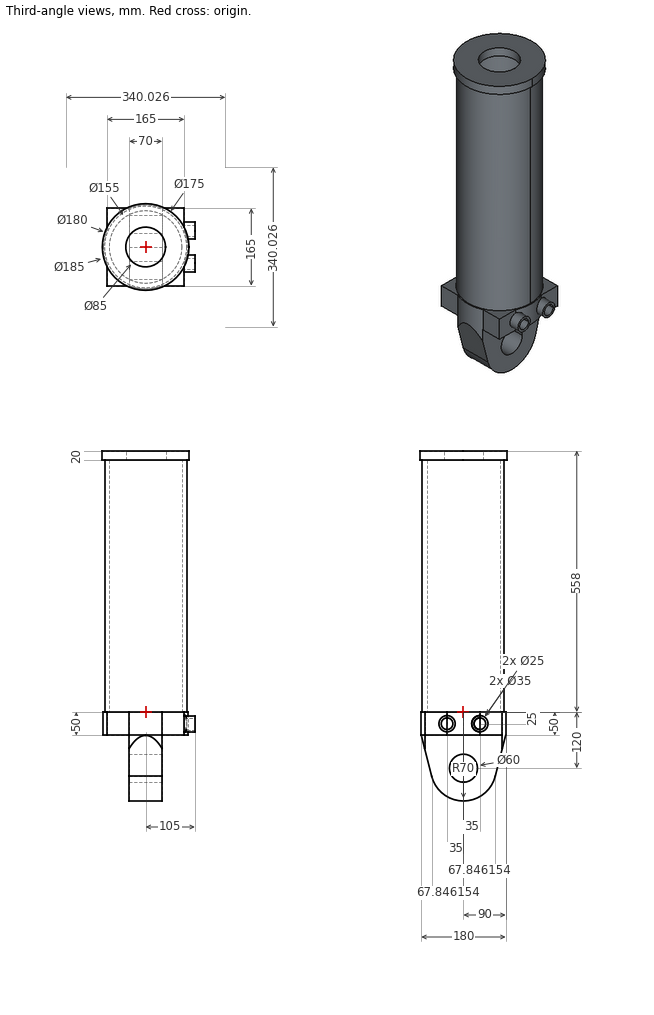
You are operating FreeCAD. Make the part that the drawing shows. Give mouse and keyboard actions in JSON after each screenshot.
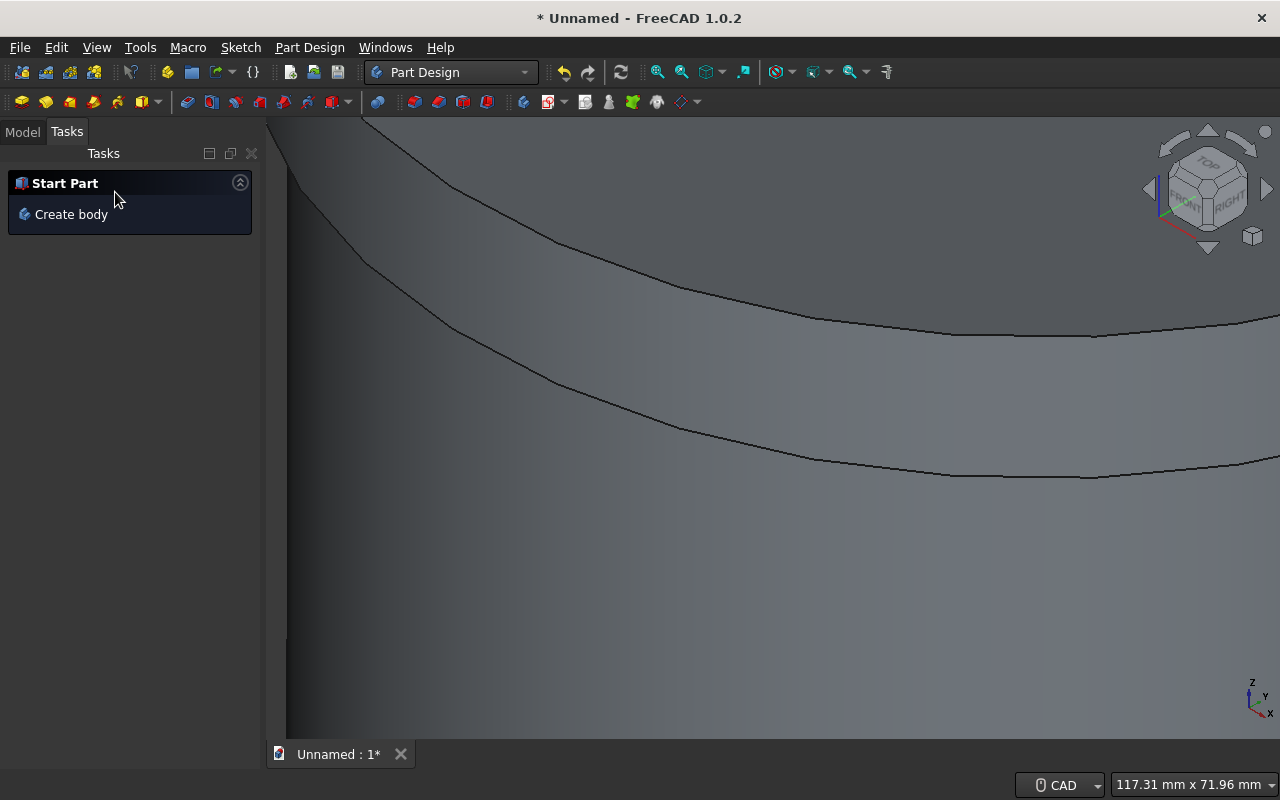
{"action": "left_click", "coordinate": [658, 72]}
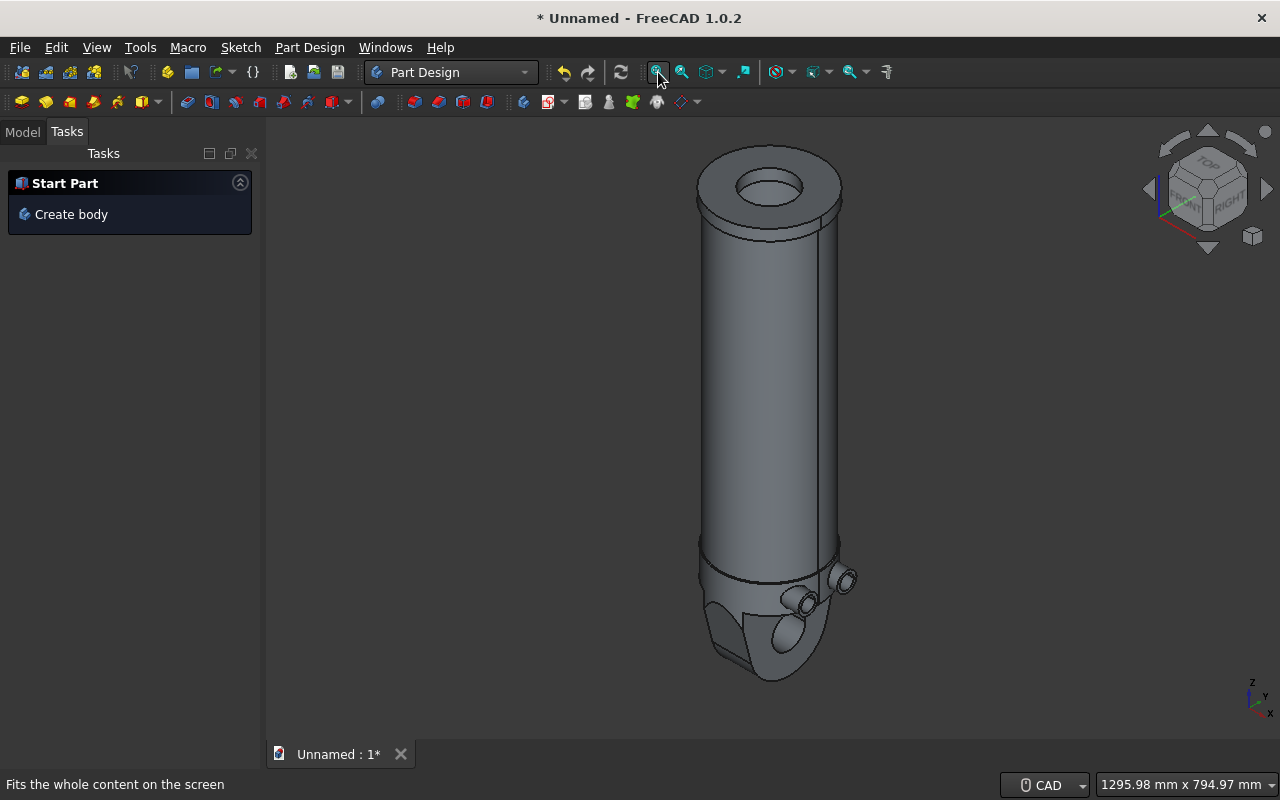
{"action": "key", "text": "5"}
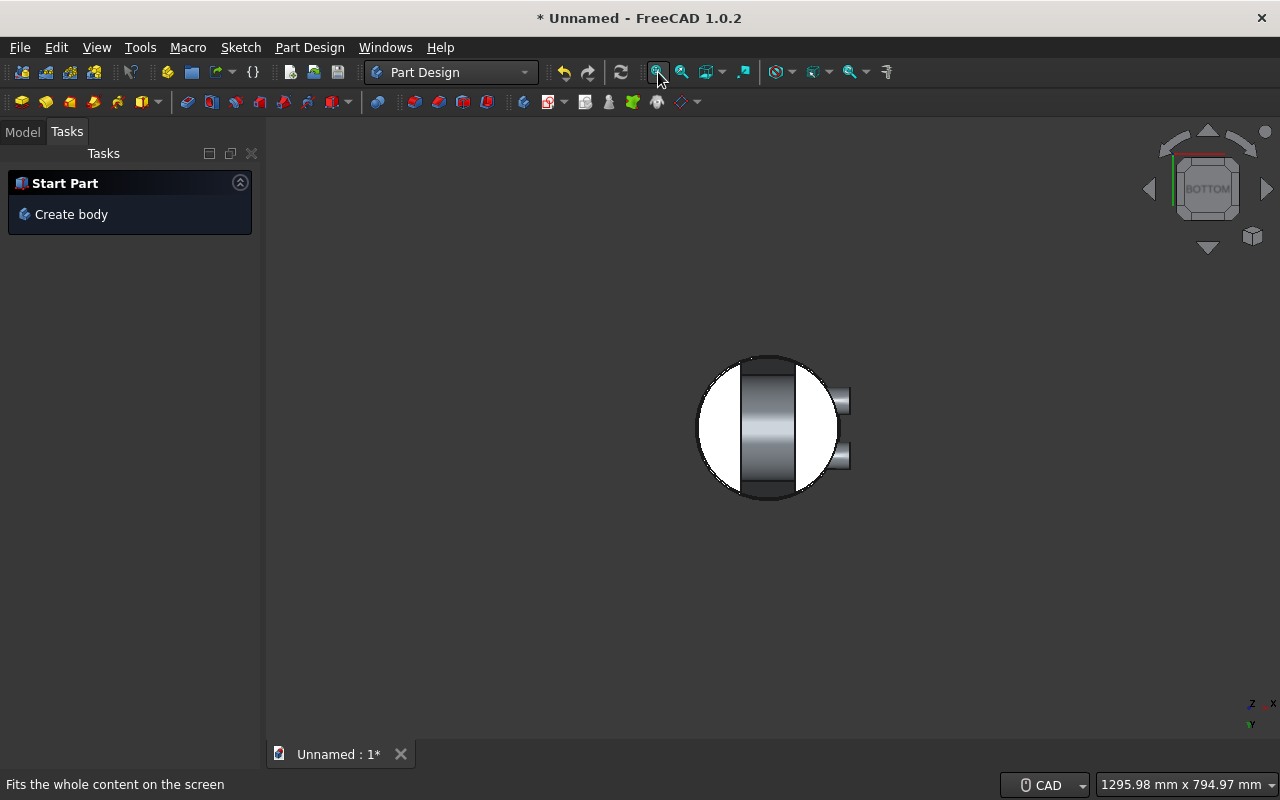
{"action": "left_click", "coordinate": [658, 72]}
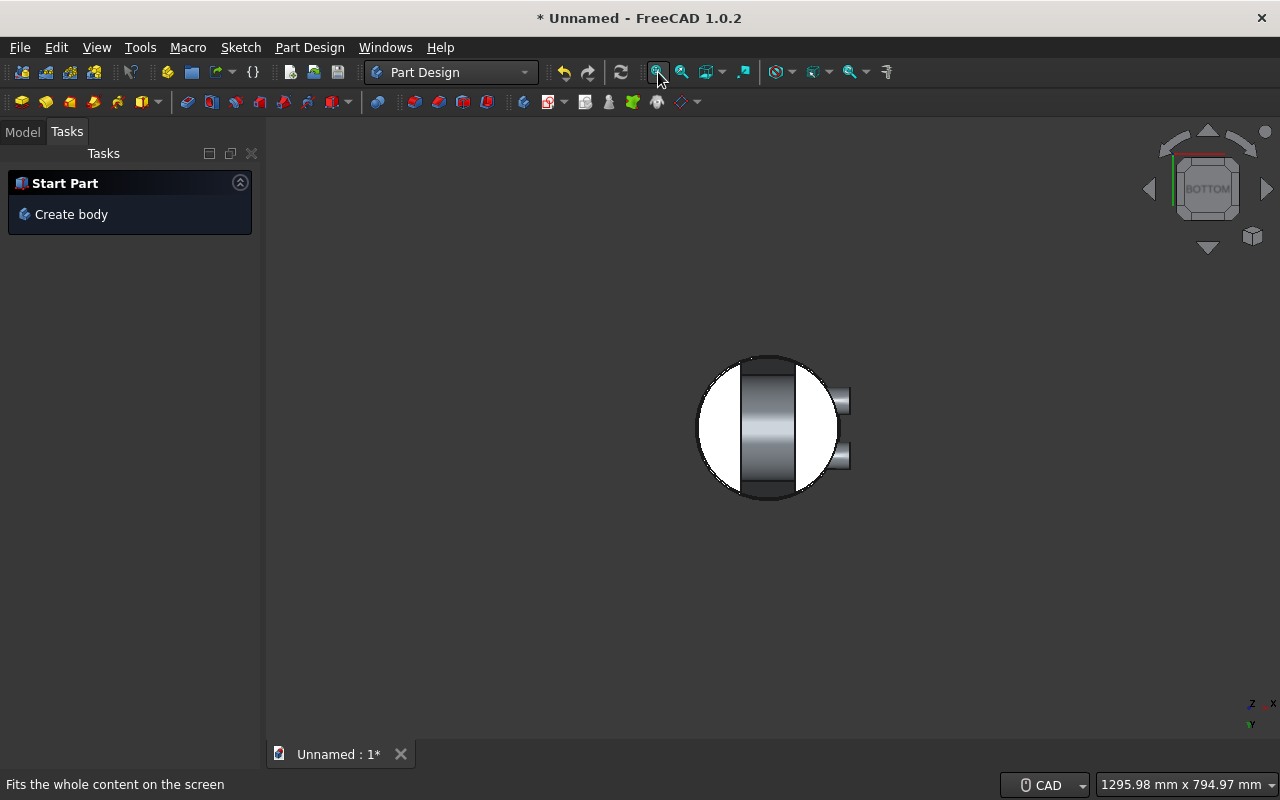
{"action": "left_click", "coordinate": [817, 427]}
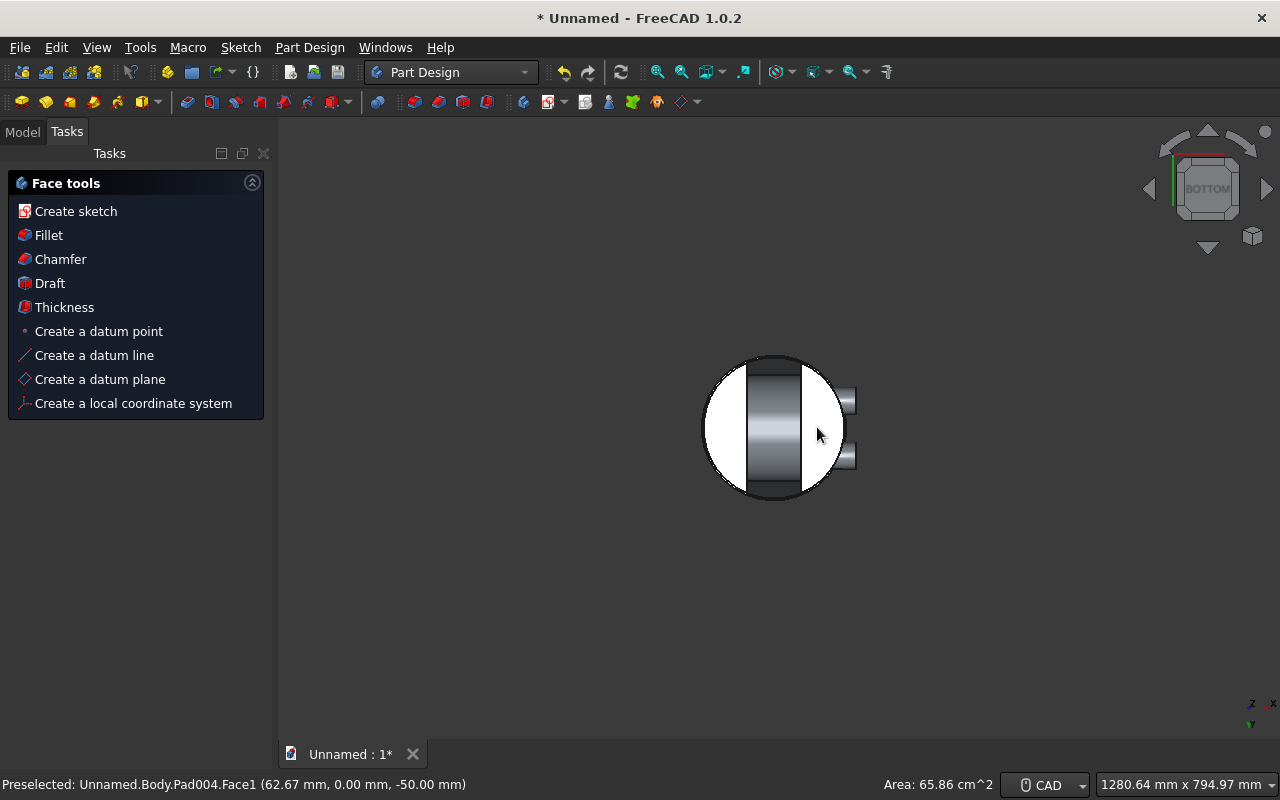
{"action": "left_click", "coordinate": [548, 102]}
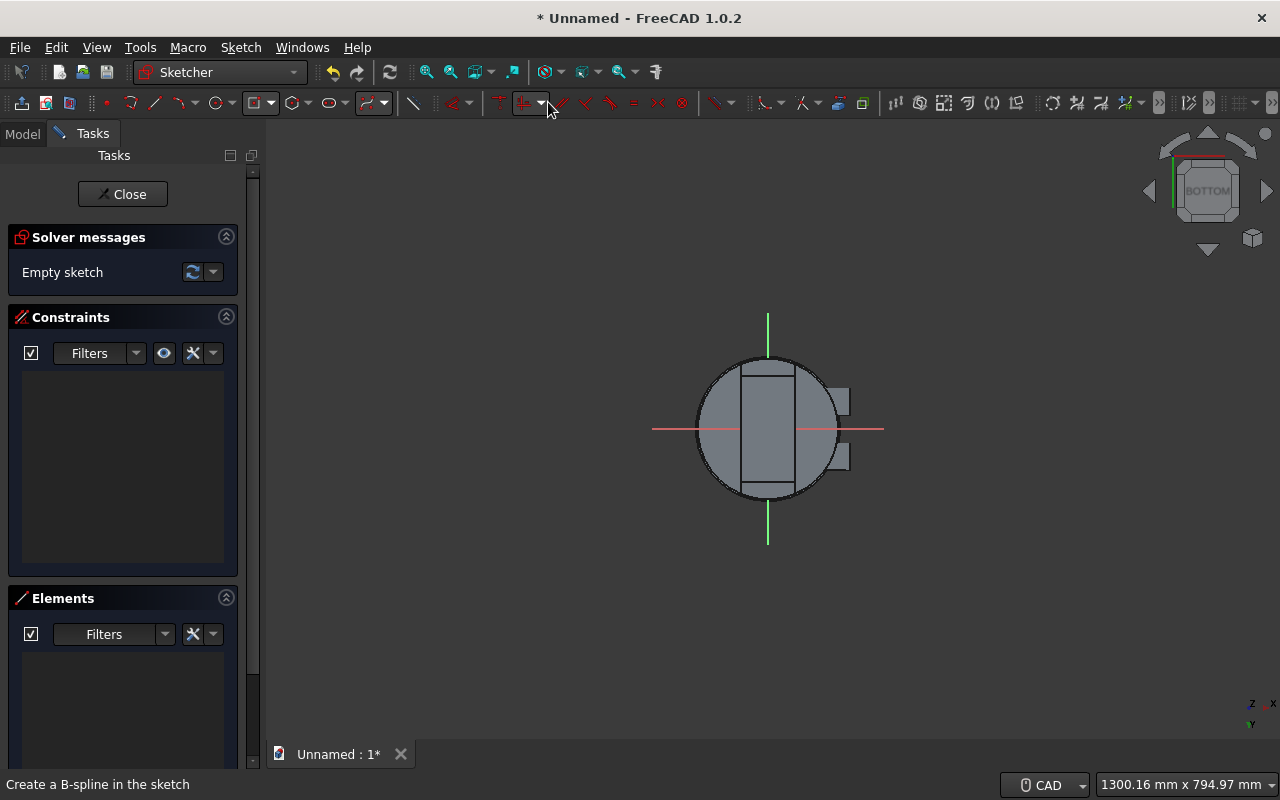
{"action": "scroll", "coordinate": [795, 429], "scroll_direction": "up", "scroll_amount": 6}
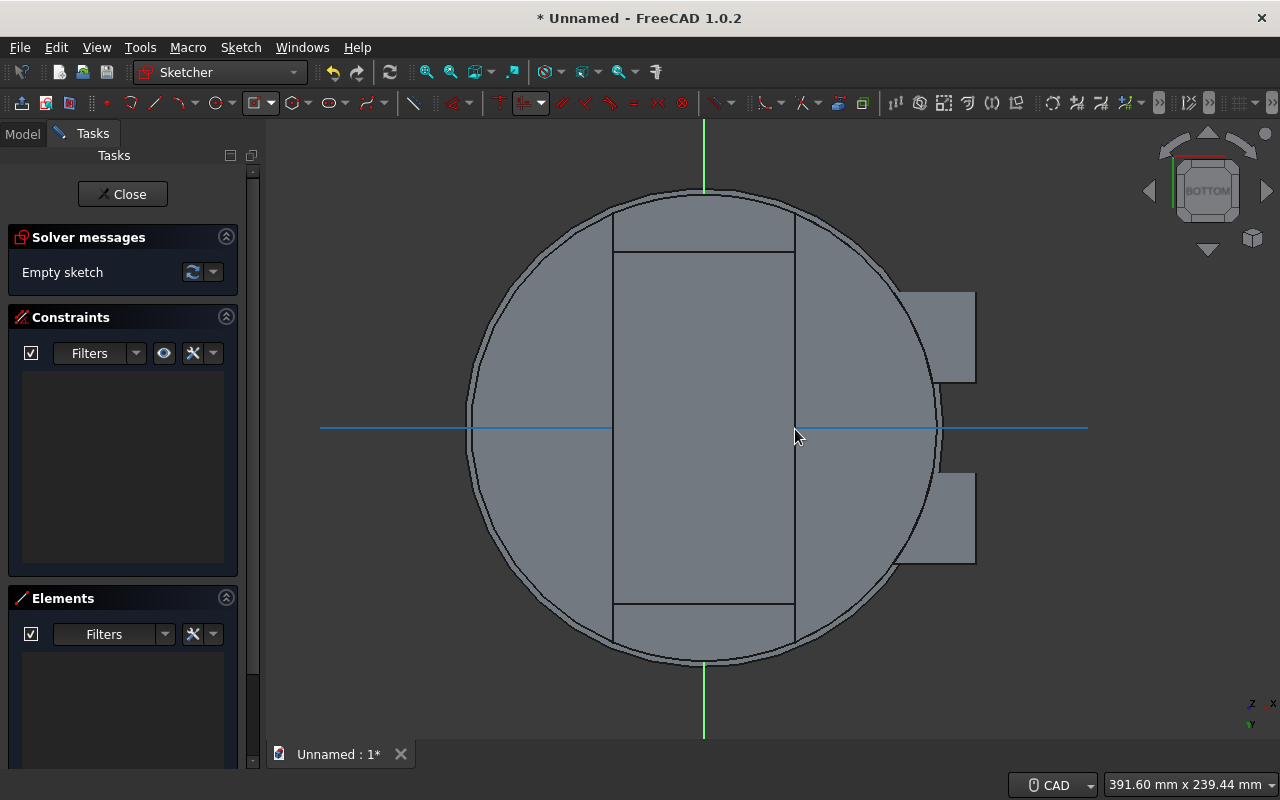
{"action": "left_click", "coordinate": [254, 104]}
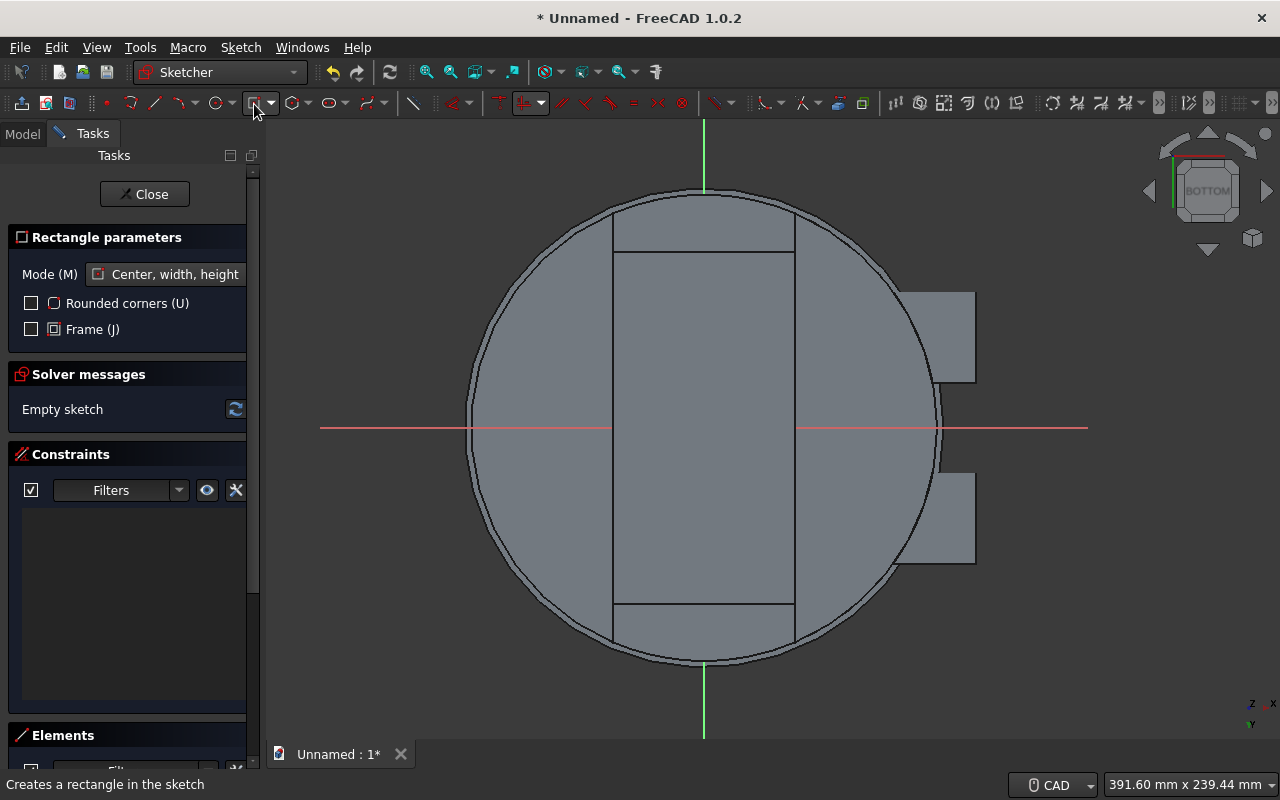
{"action": "left_click", "coordinate": [704, 428]}
{"action": "left_click", "coordinate": [918, 214]}
{"action": "key", "text": "Escape"}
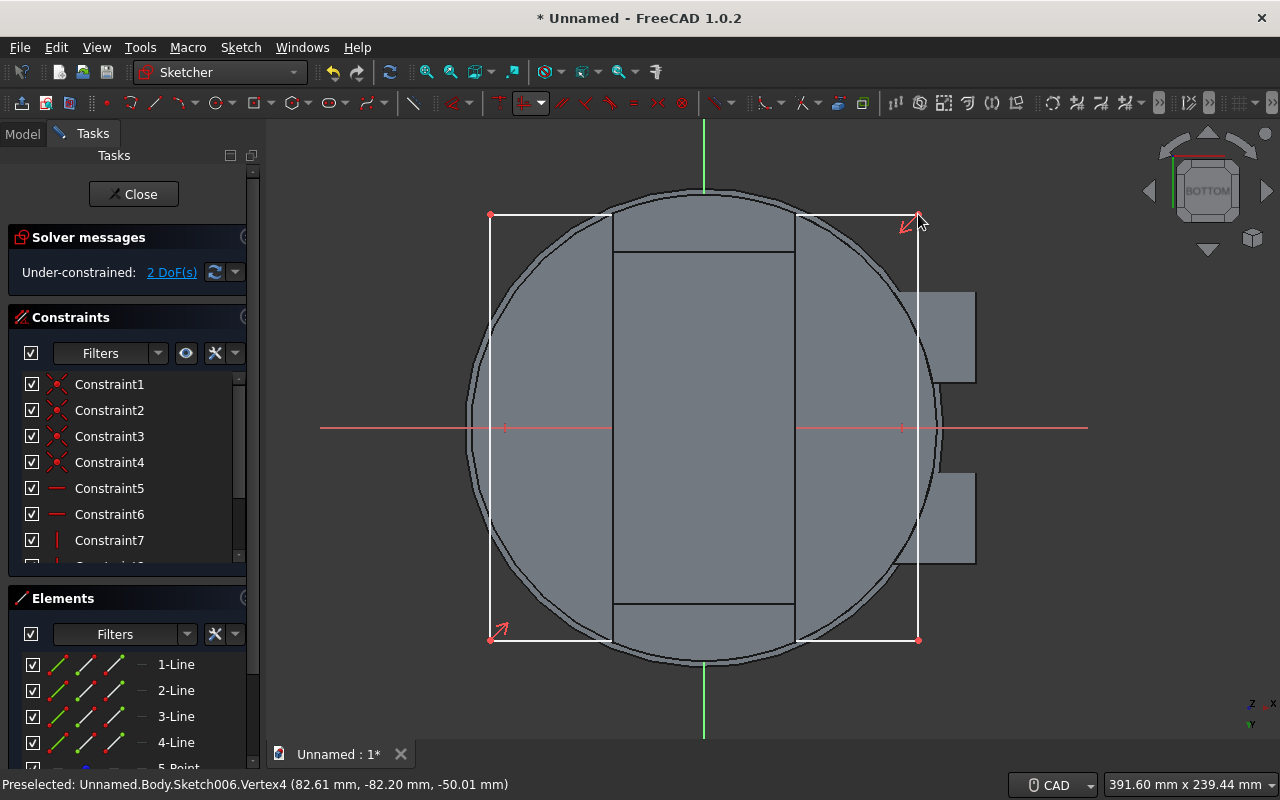
{"action": "left_click", "coordinate": [452, 104]}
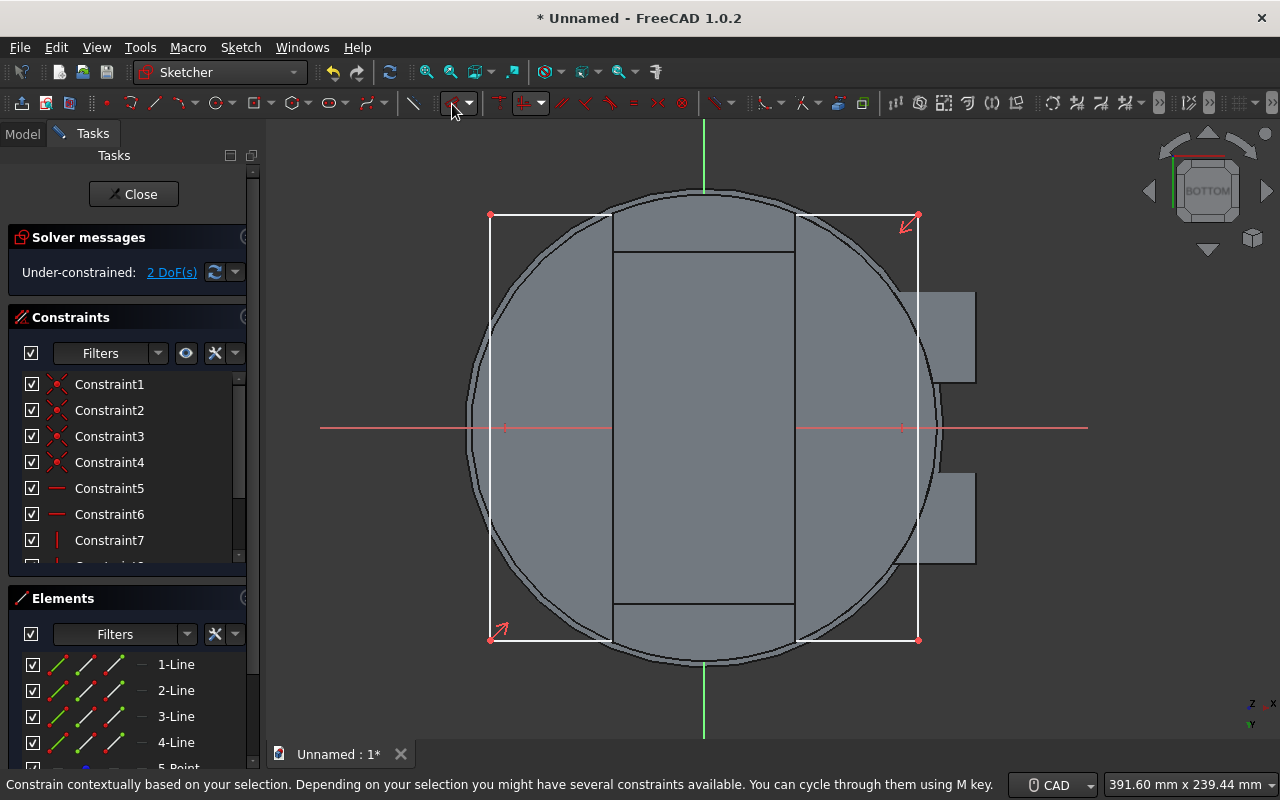
{"action": "left_click", "coordinate": [619, 641]}
{"action": "left_click", "coordinate": [606, 675]}